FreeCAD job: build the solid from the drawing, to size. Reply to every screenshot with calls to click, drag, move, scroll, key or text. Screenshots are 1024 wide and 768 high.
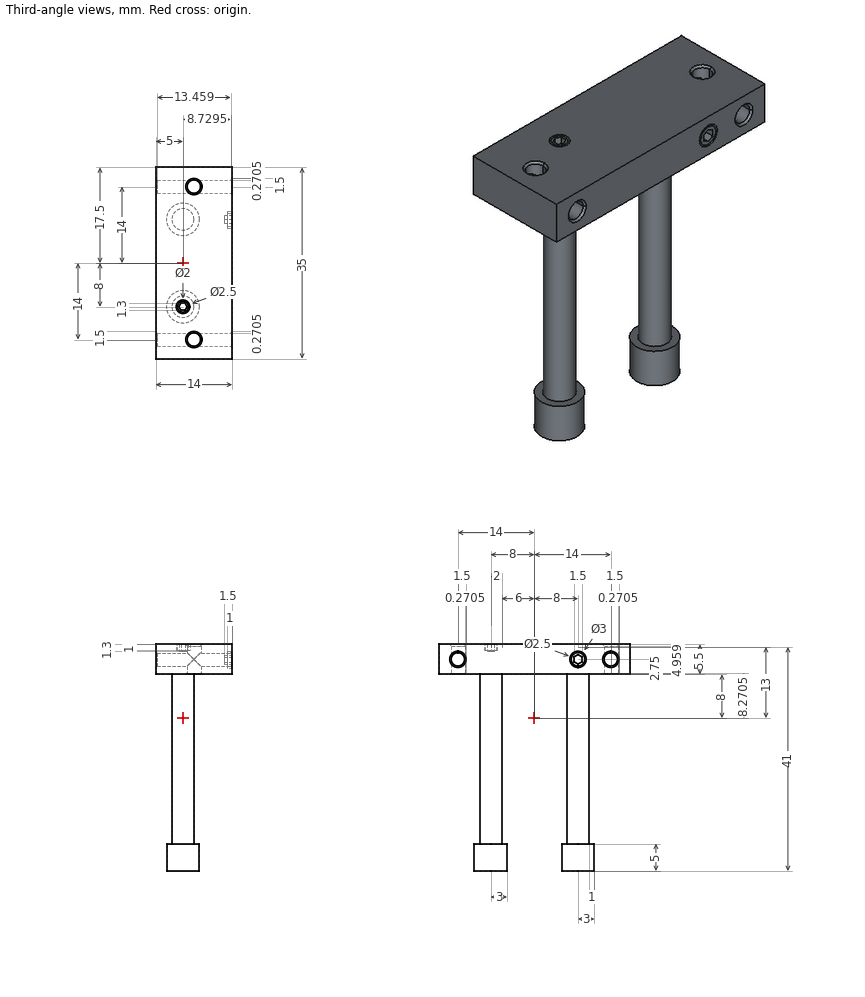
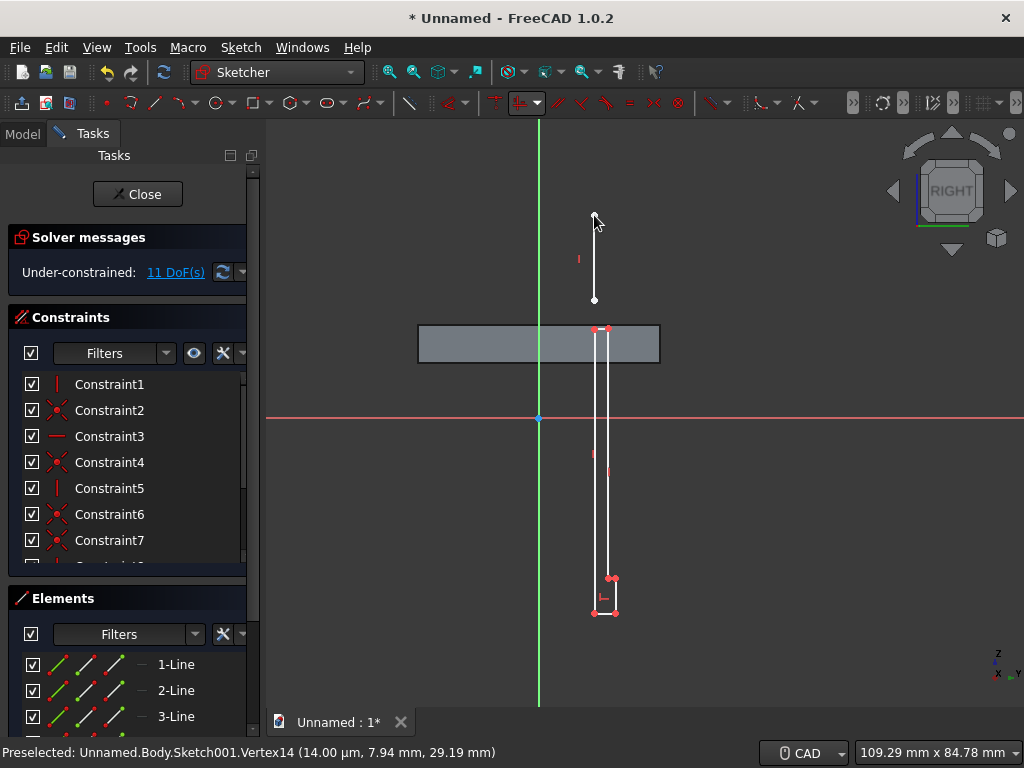
click(594, 276)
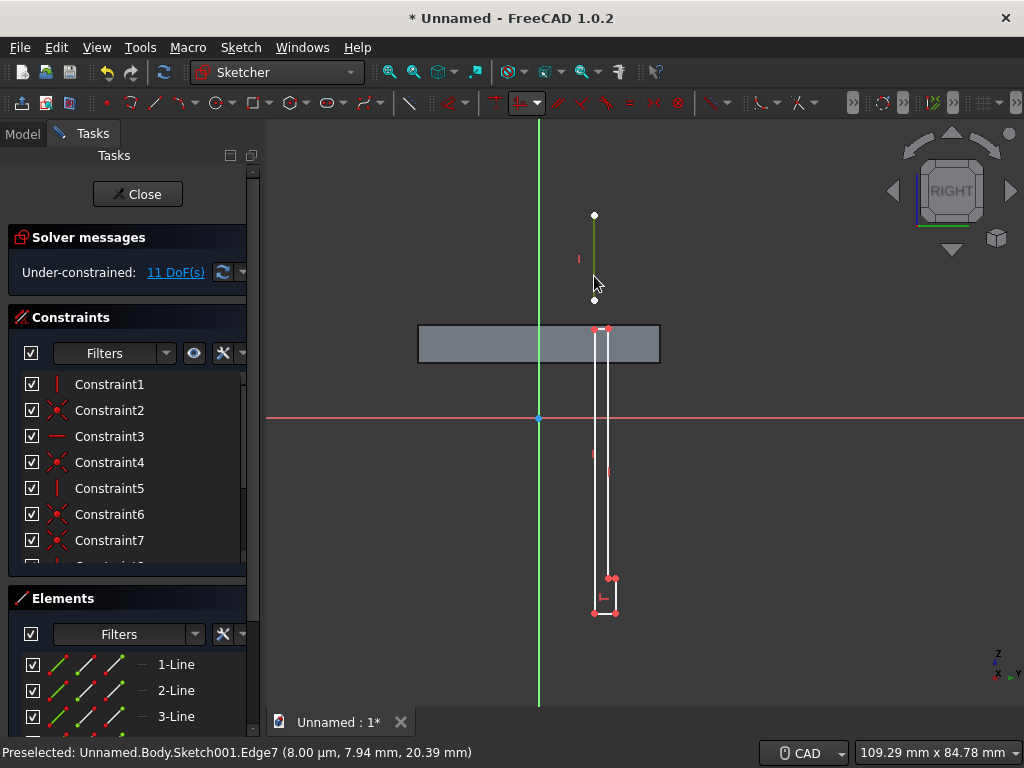
click(410, 104)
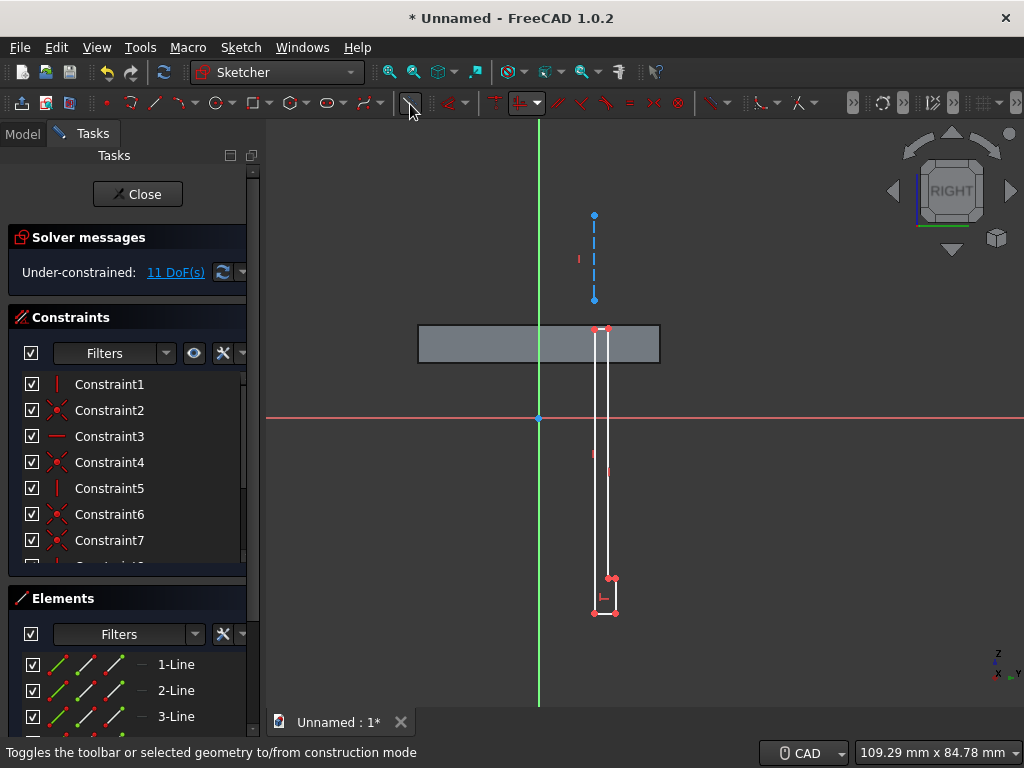
scroll(612, 578, up, 7)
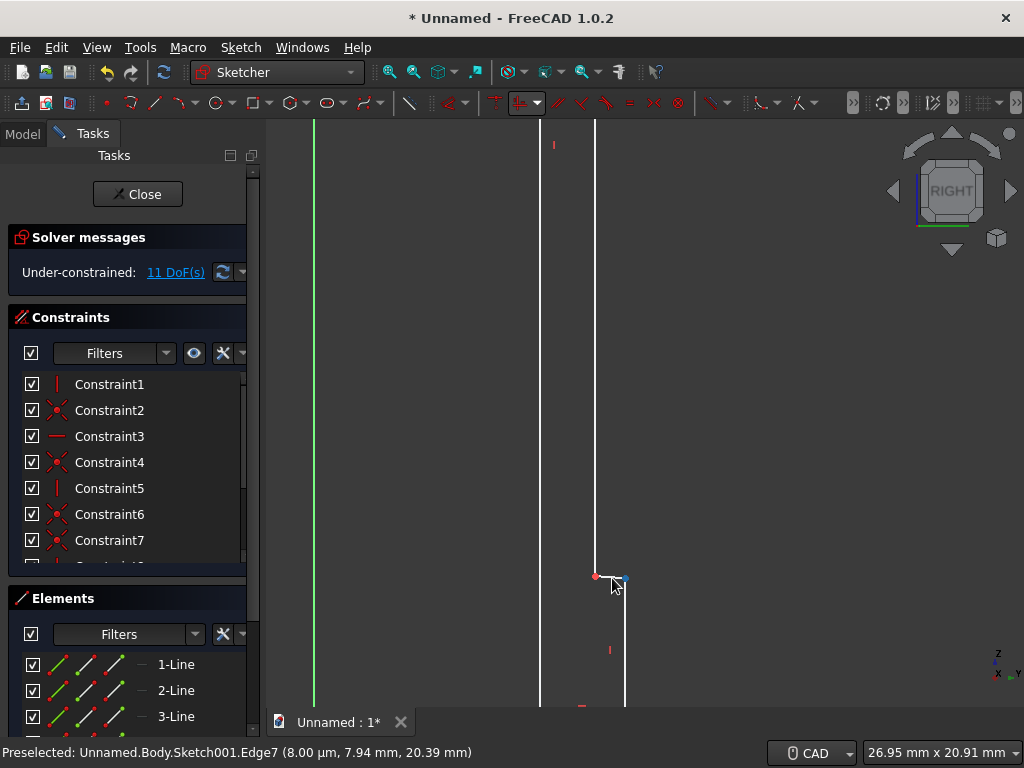
click(610, 577)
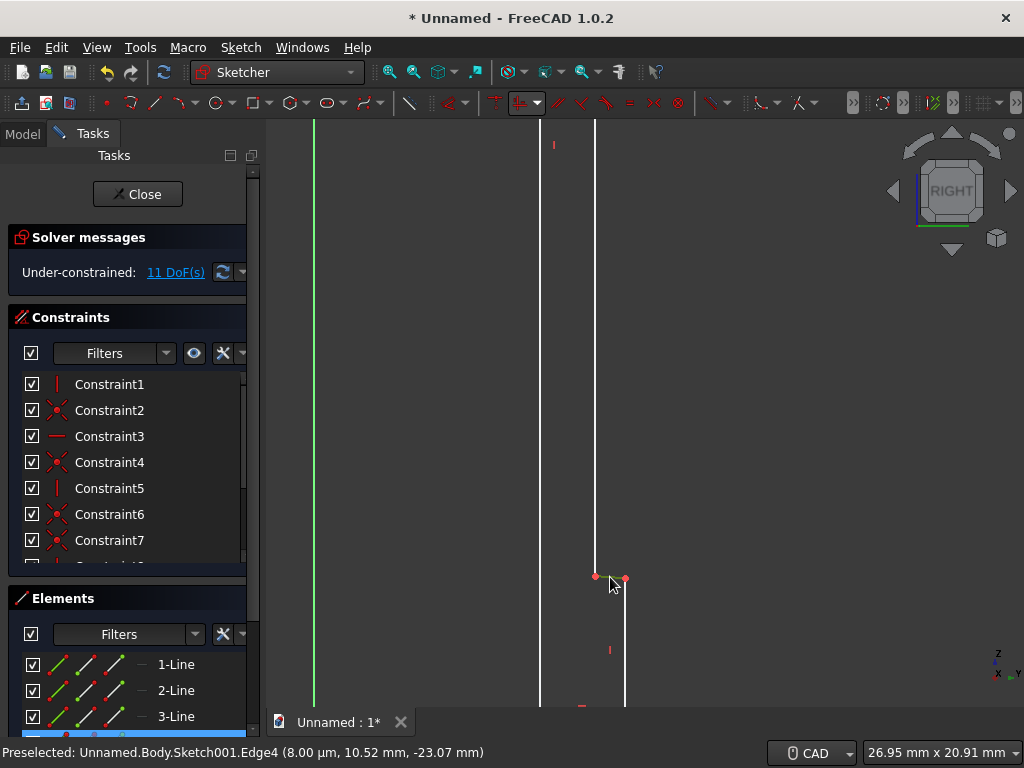
click(540, 104)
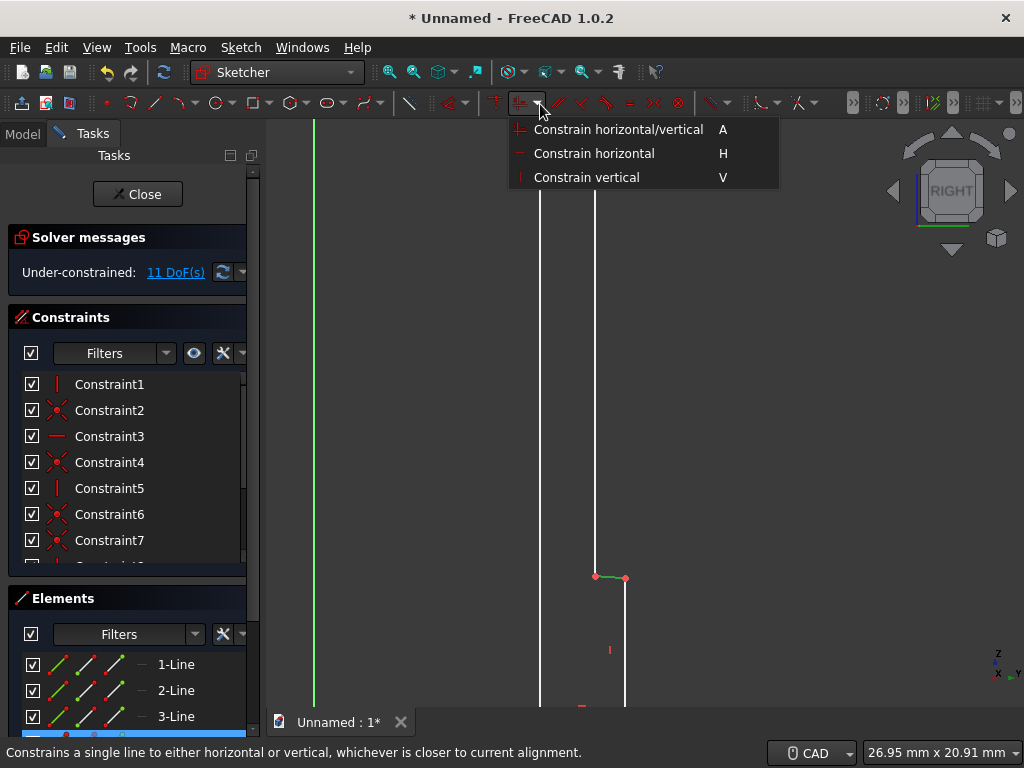
click(644, 153)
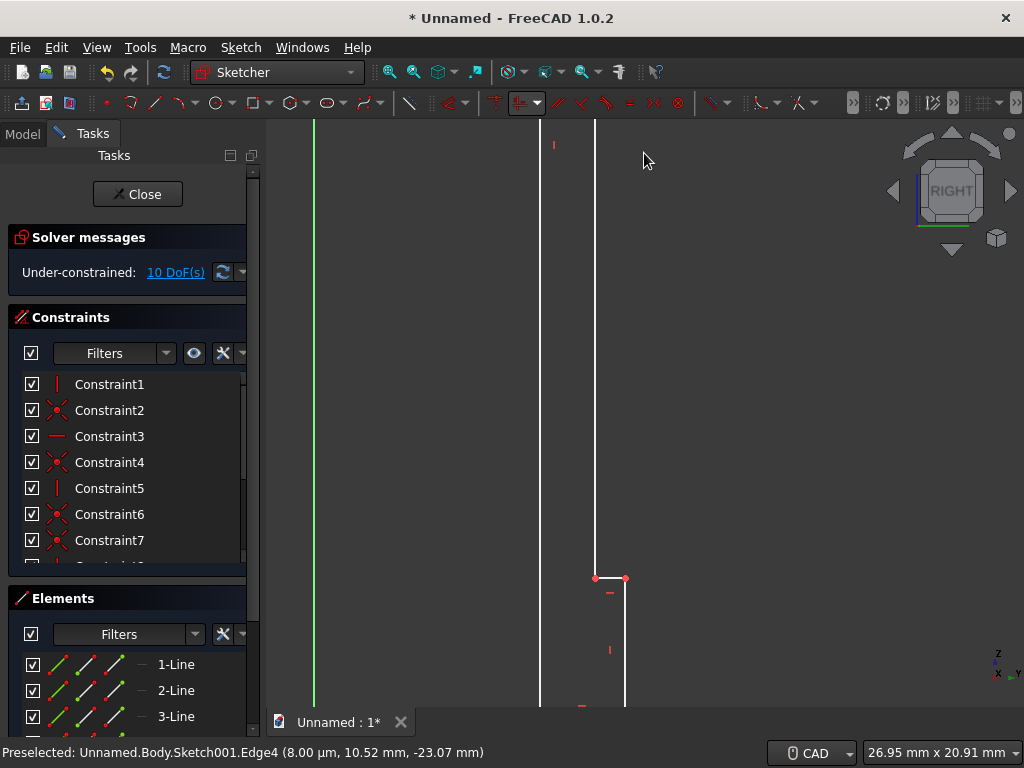
scroll(612, 578, down, 7)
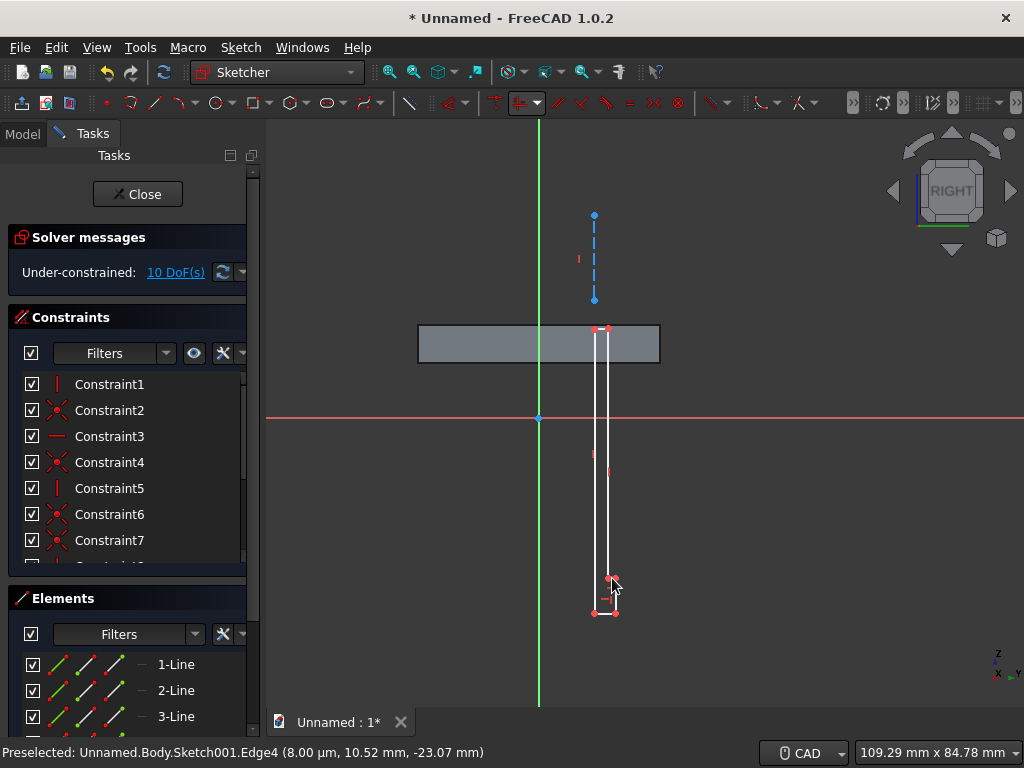
scroll(604, 329, up, 7)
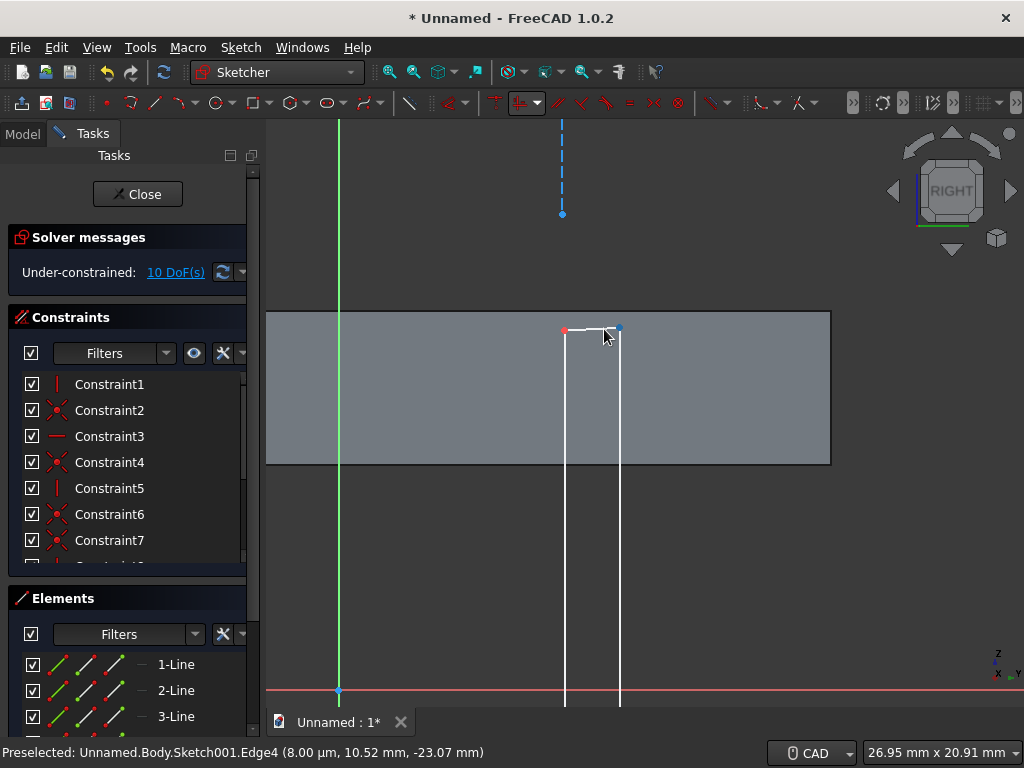
click(603, 329)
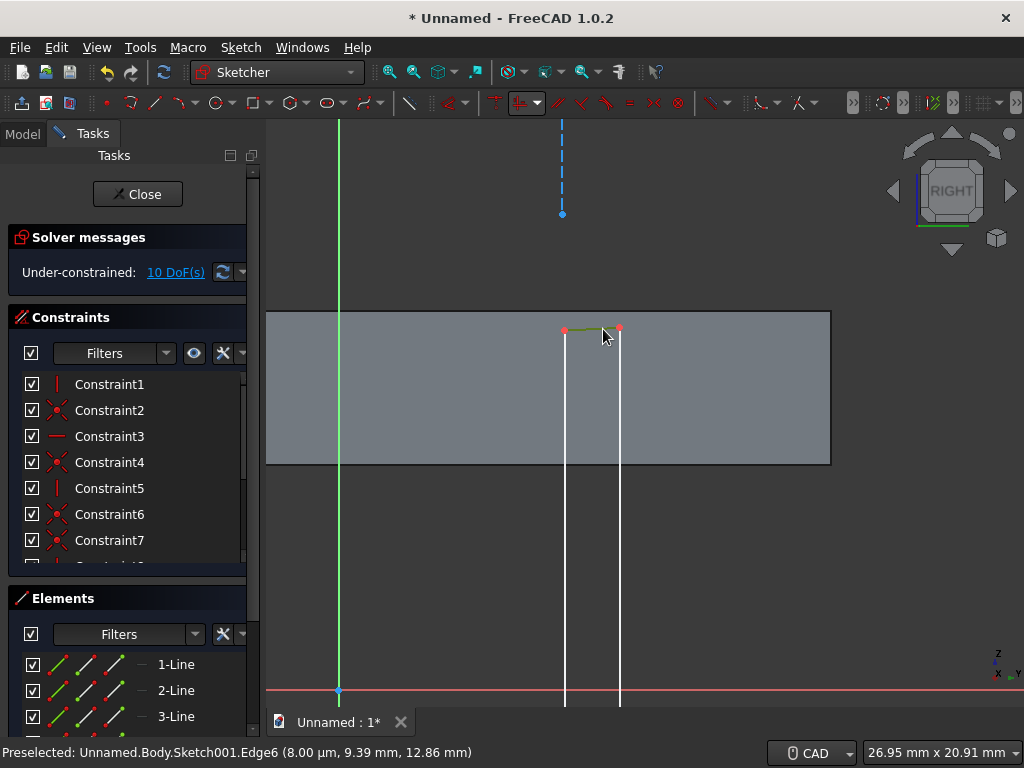
click(540, 104)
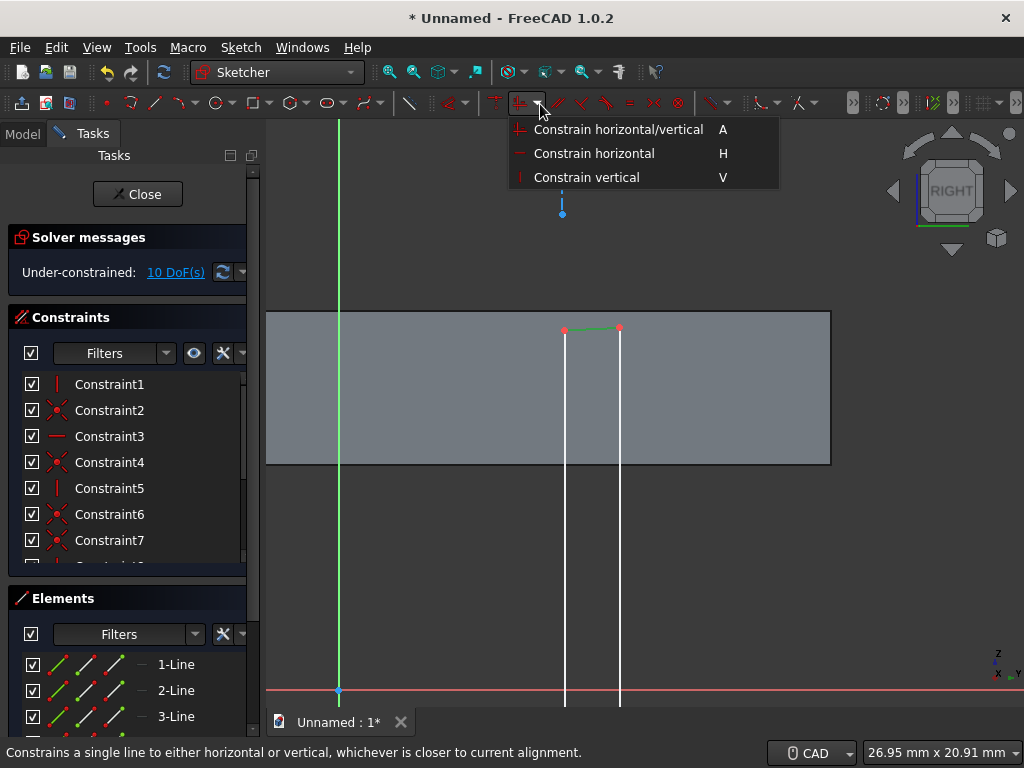
click(644, 153)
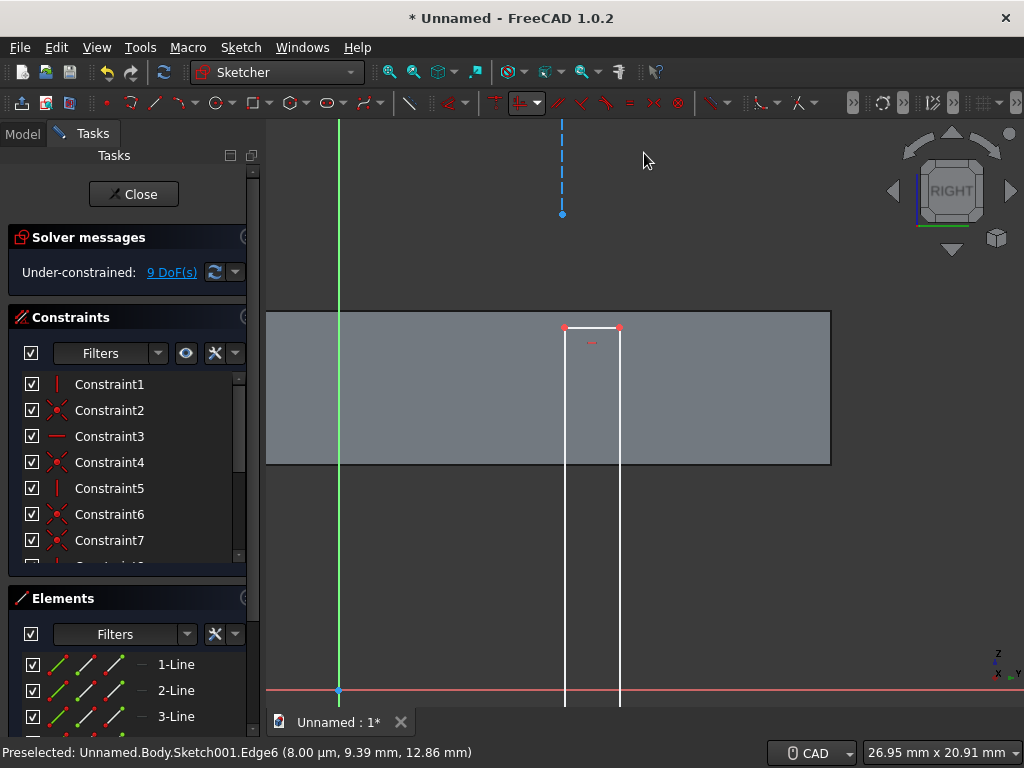
click(448, 104)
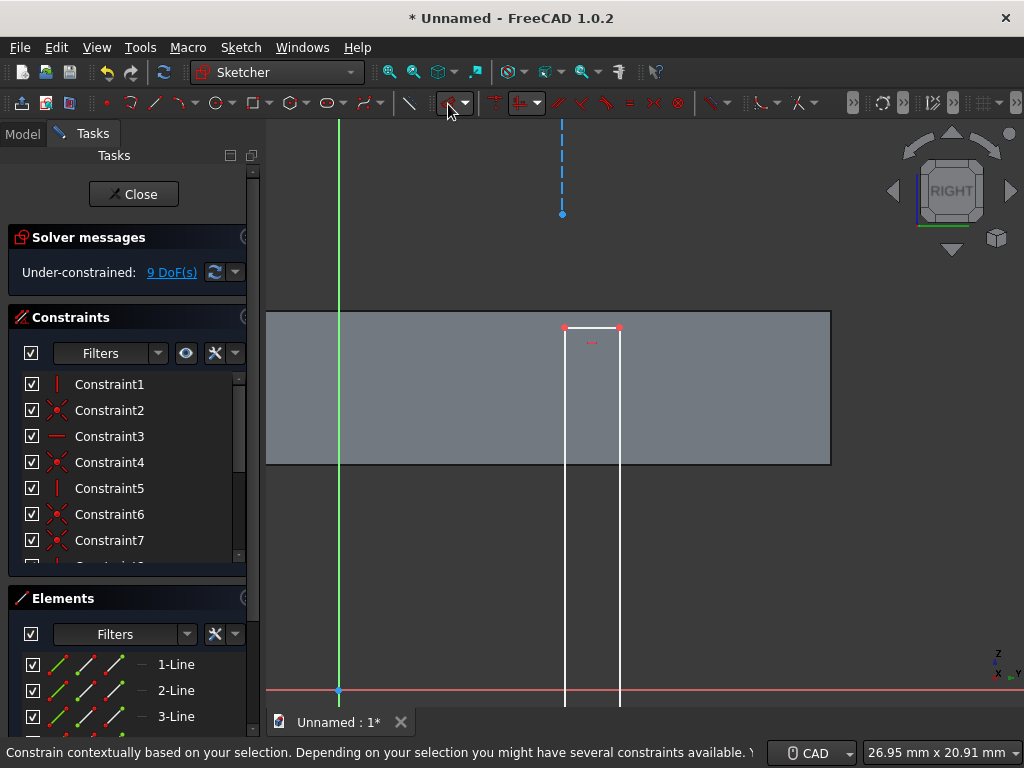
scroll(604, 329, down, 7)